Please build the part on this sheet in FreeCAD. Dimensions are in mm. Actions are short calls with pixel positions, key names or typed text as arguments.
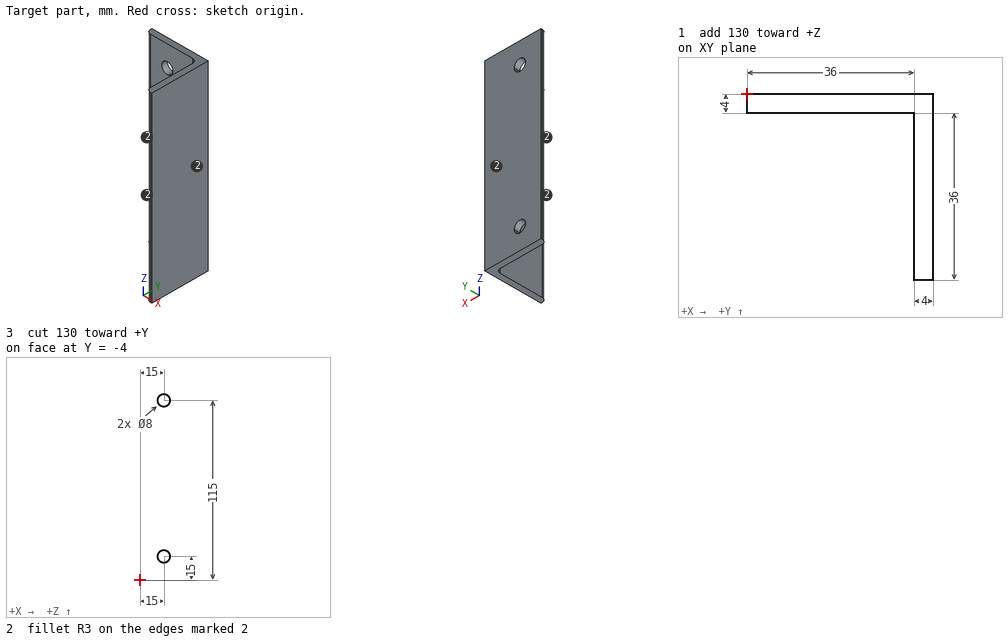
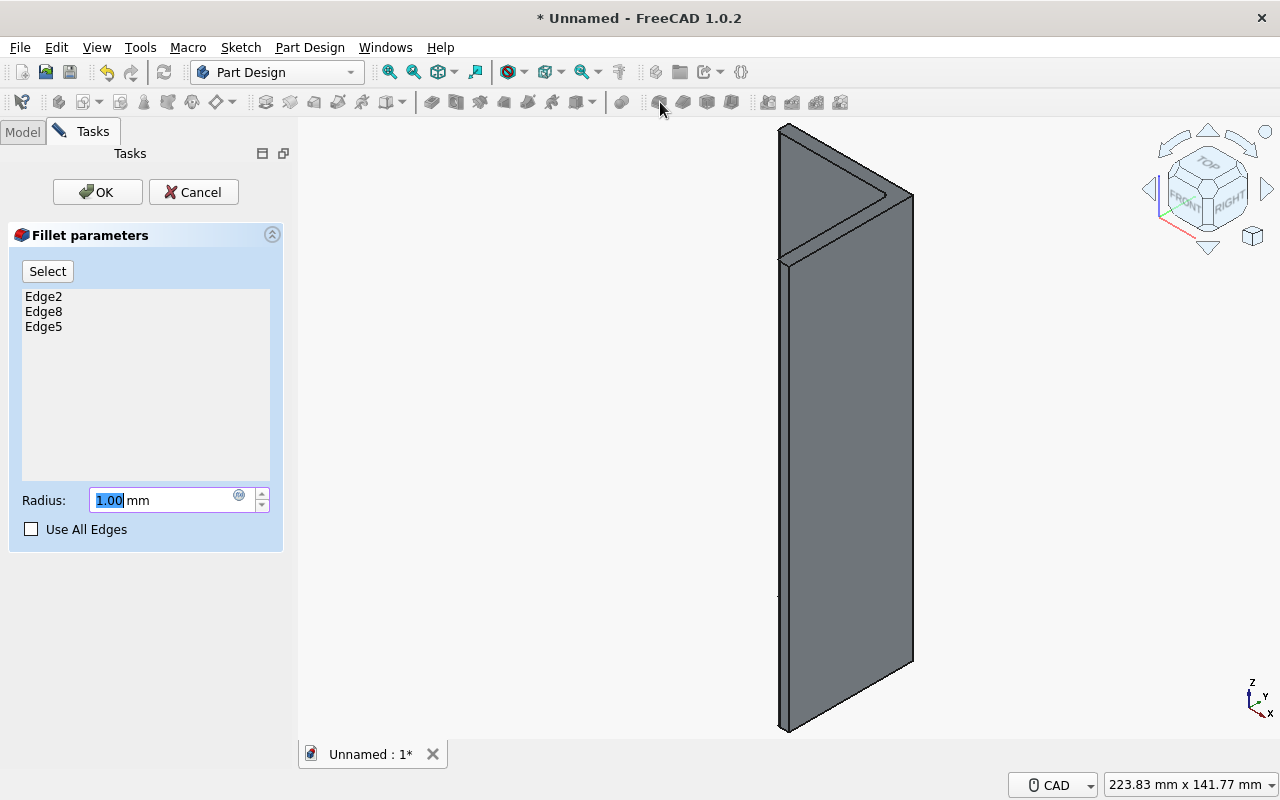
text(3)
key(Tab)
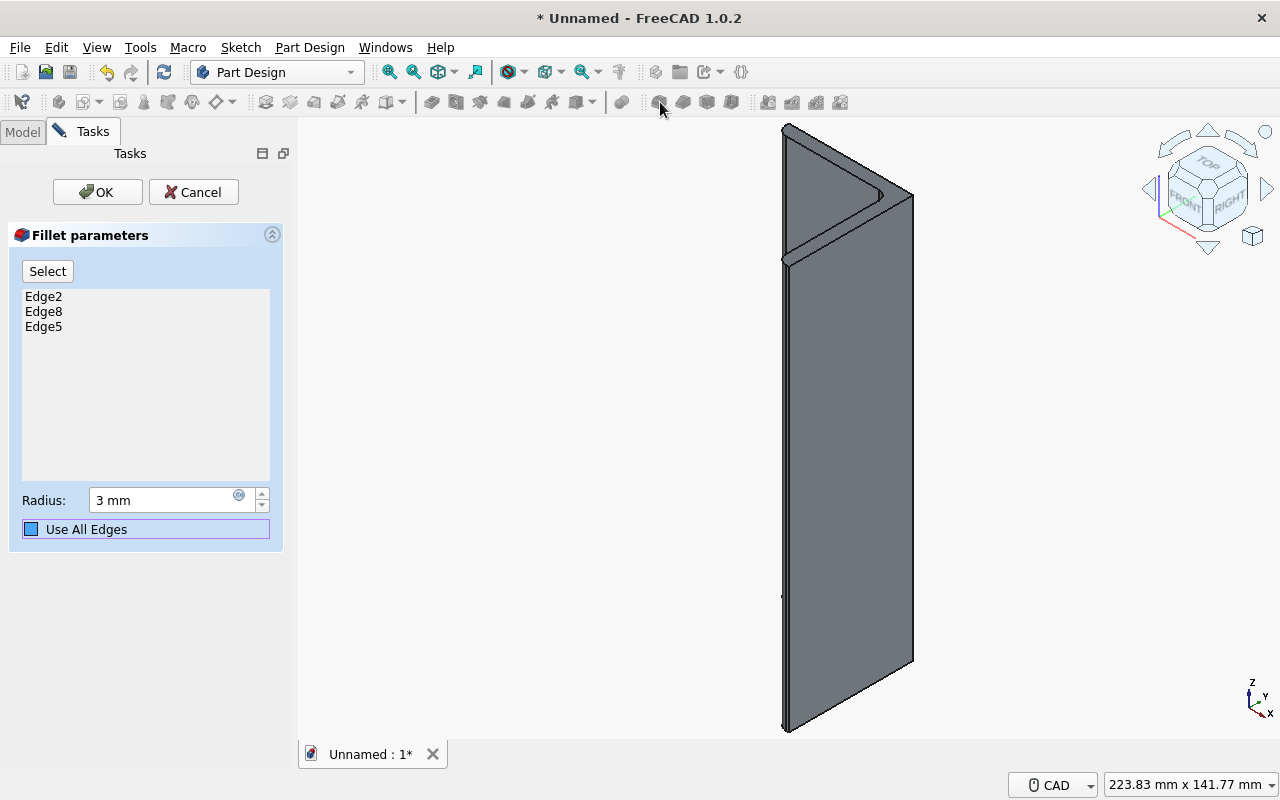
click(98, 192)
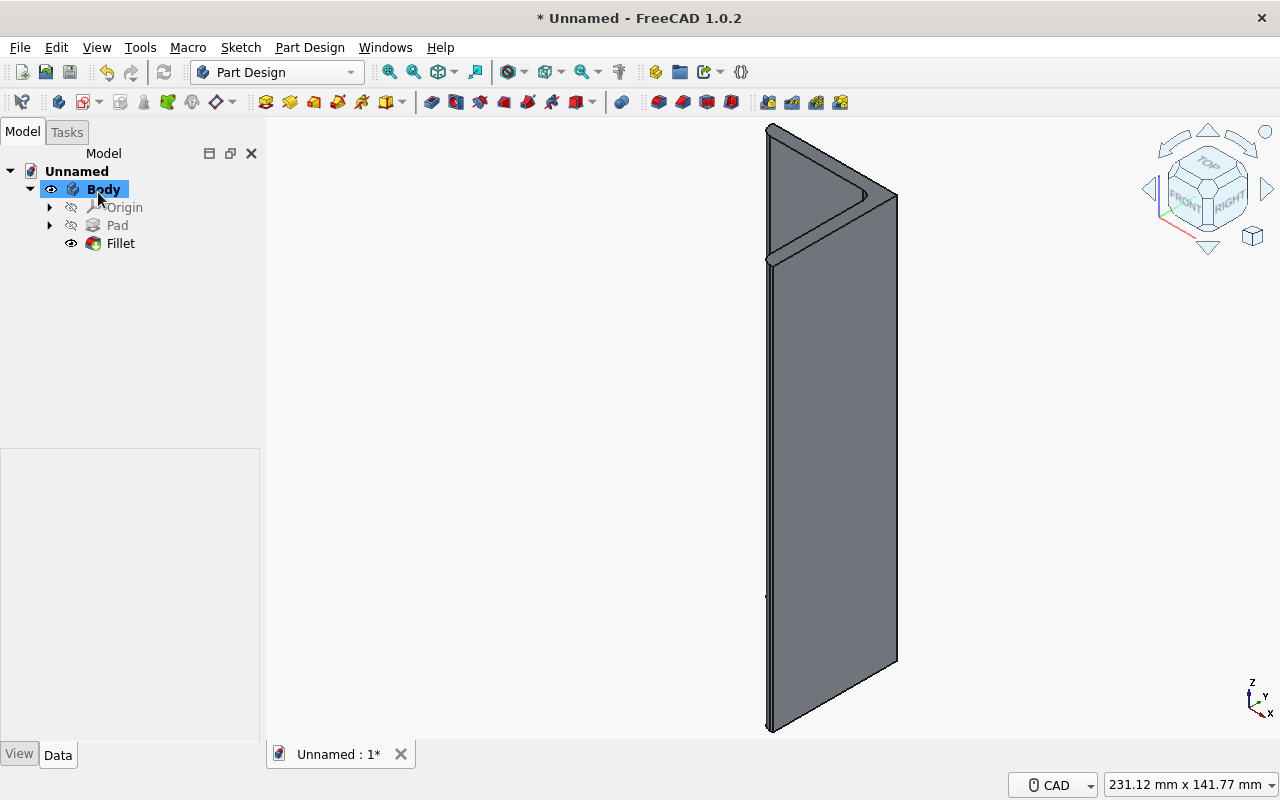
key(1)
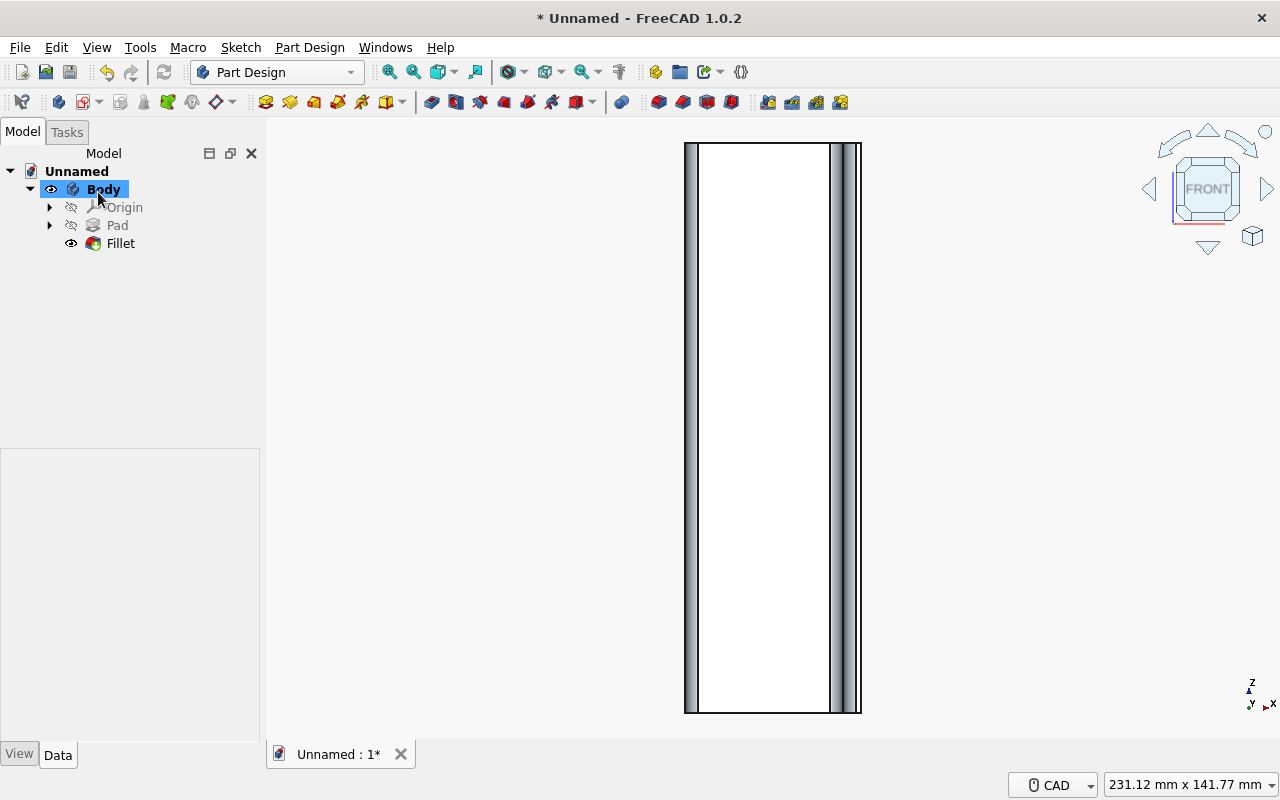
click(764, 264)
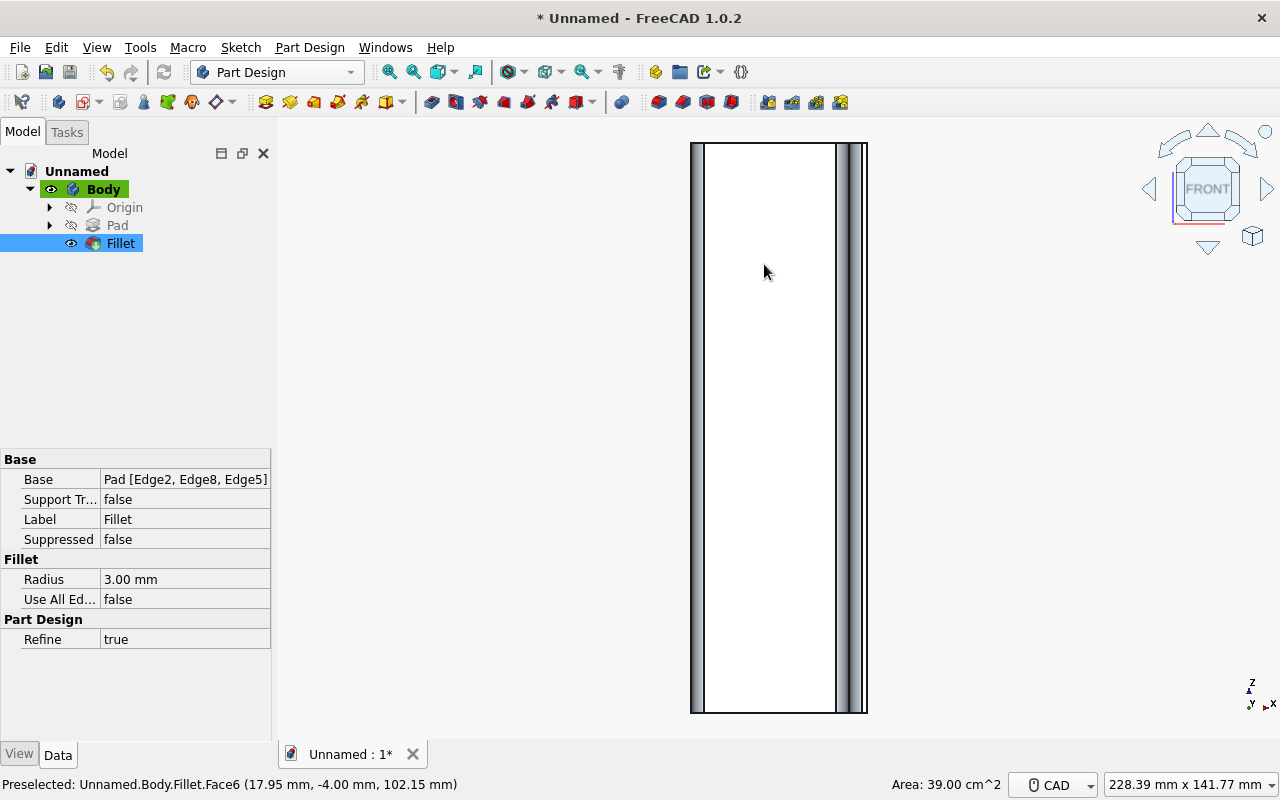
click(84, 102)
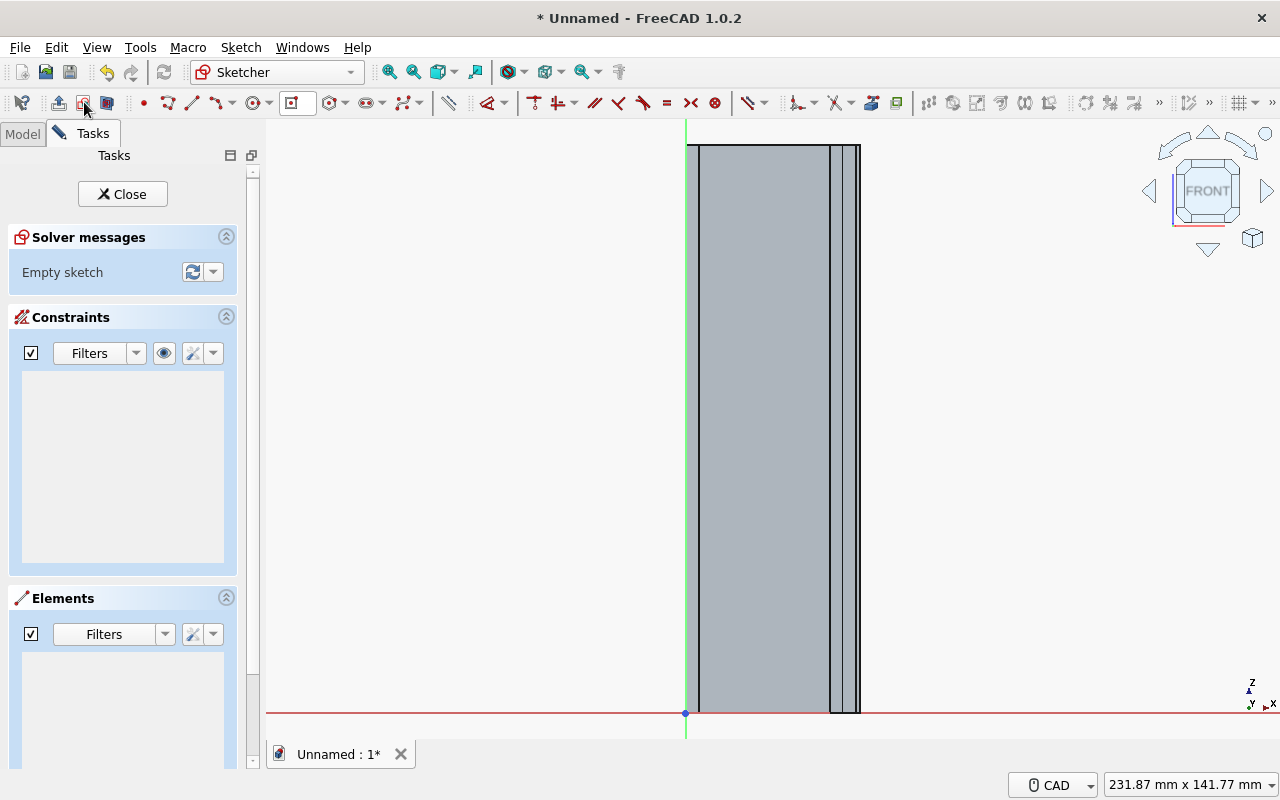
scroll(603, 320, down, 1)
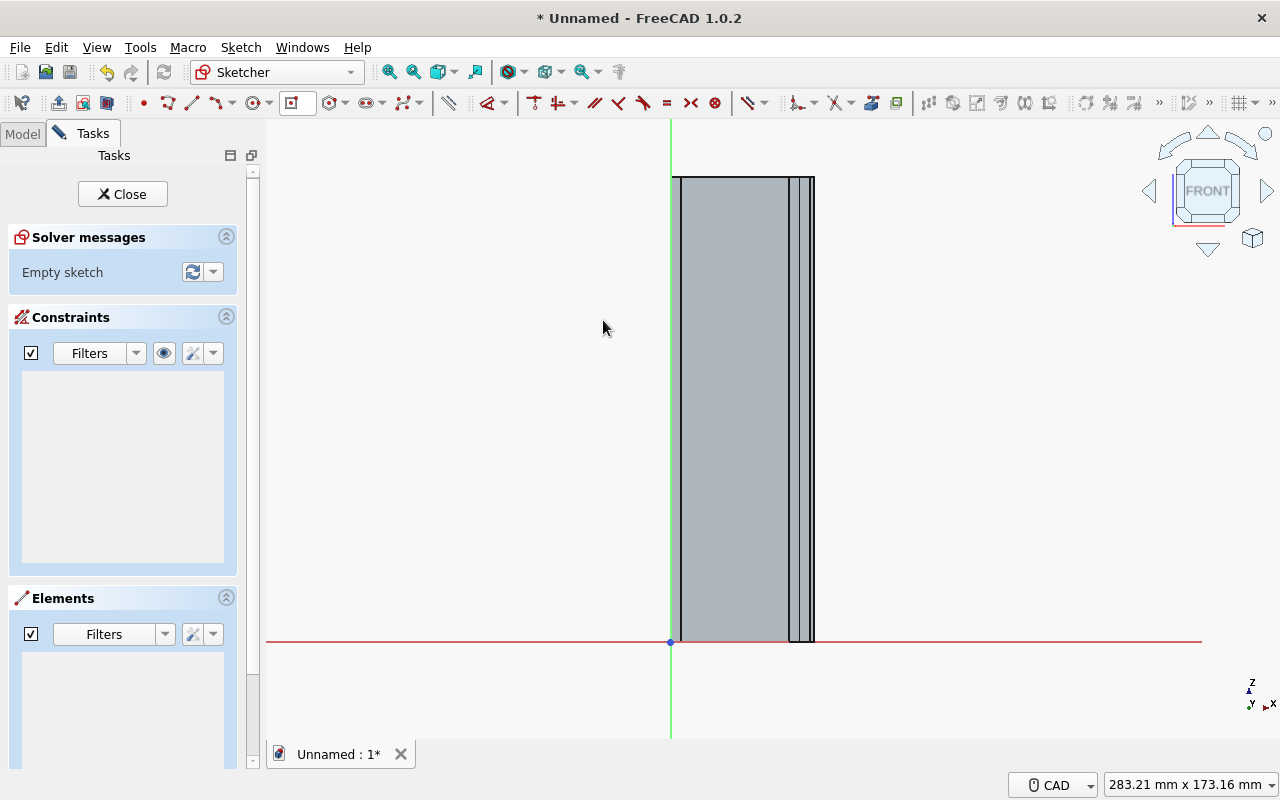
click(254, 104)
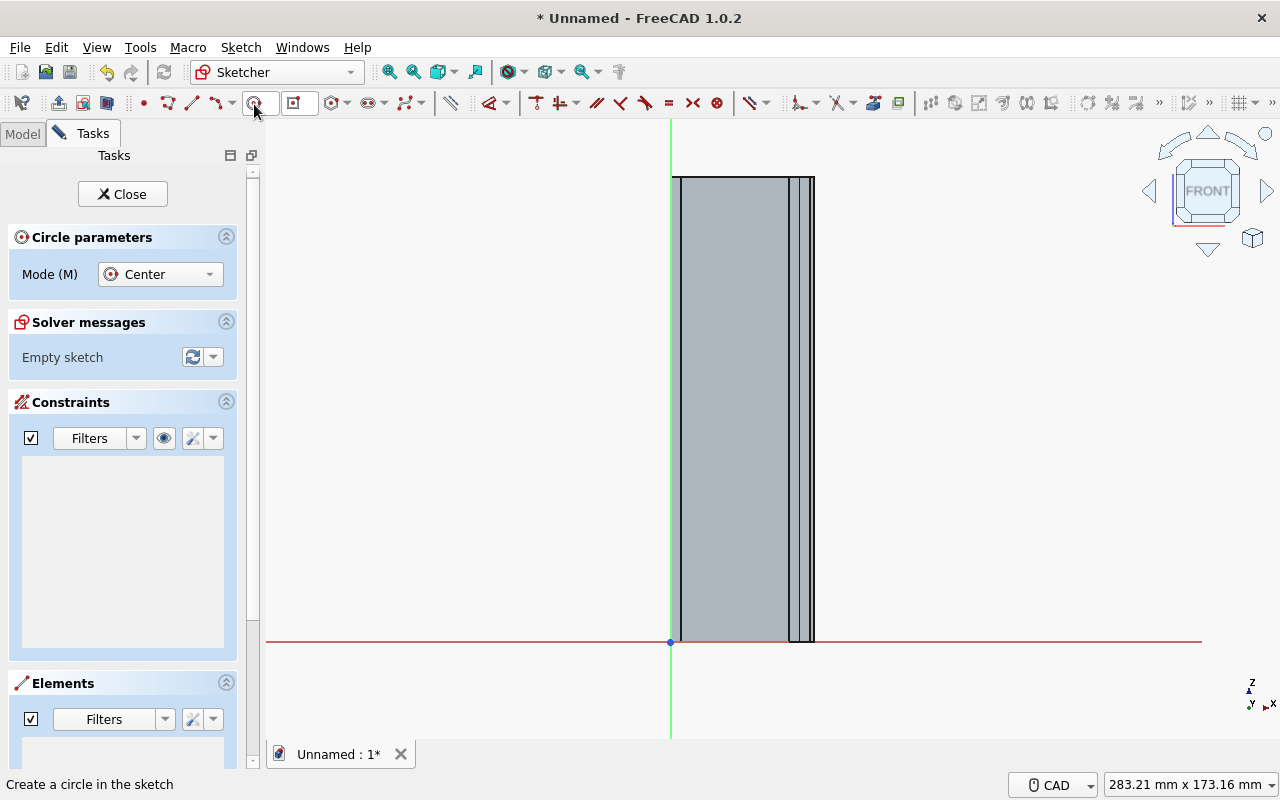
scroll(724, 230, up, 3)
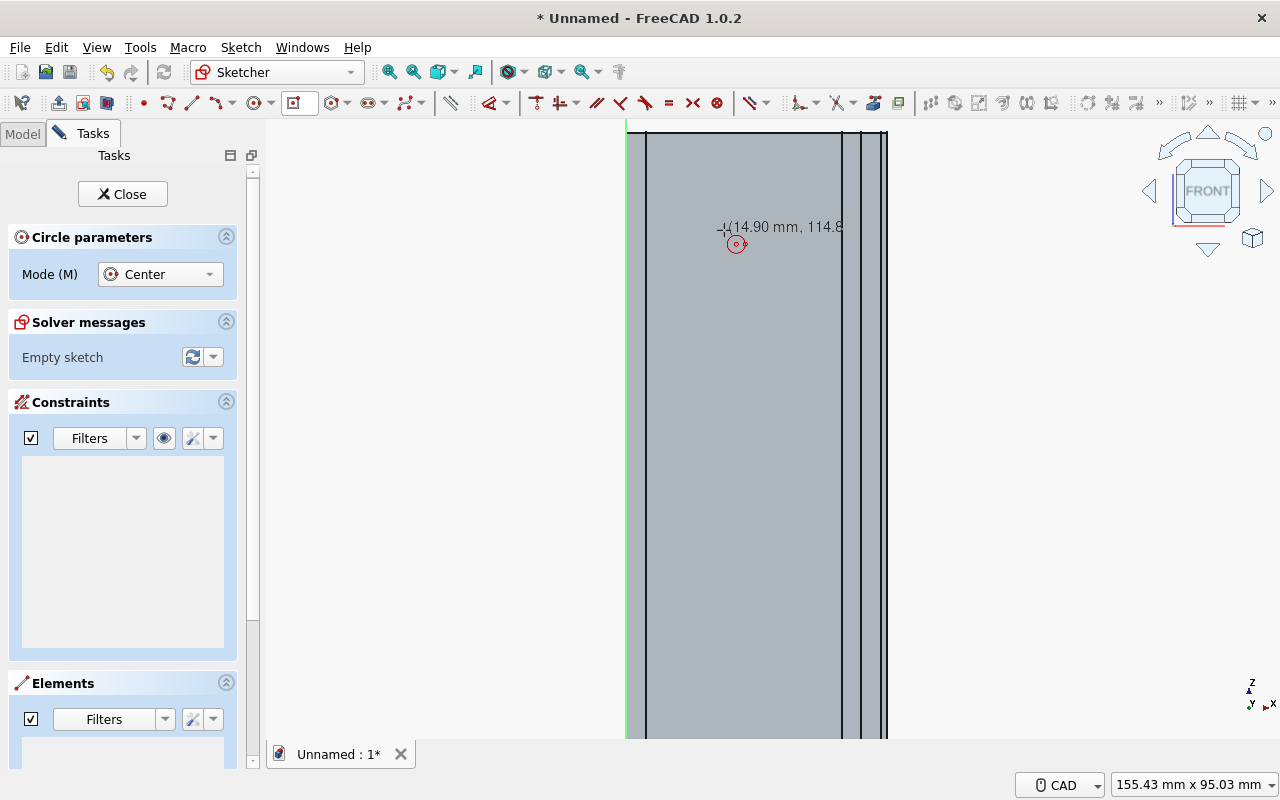
click(724, 230)
move(743, 212)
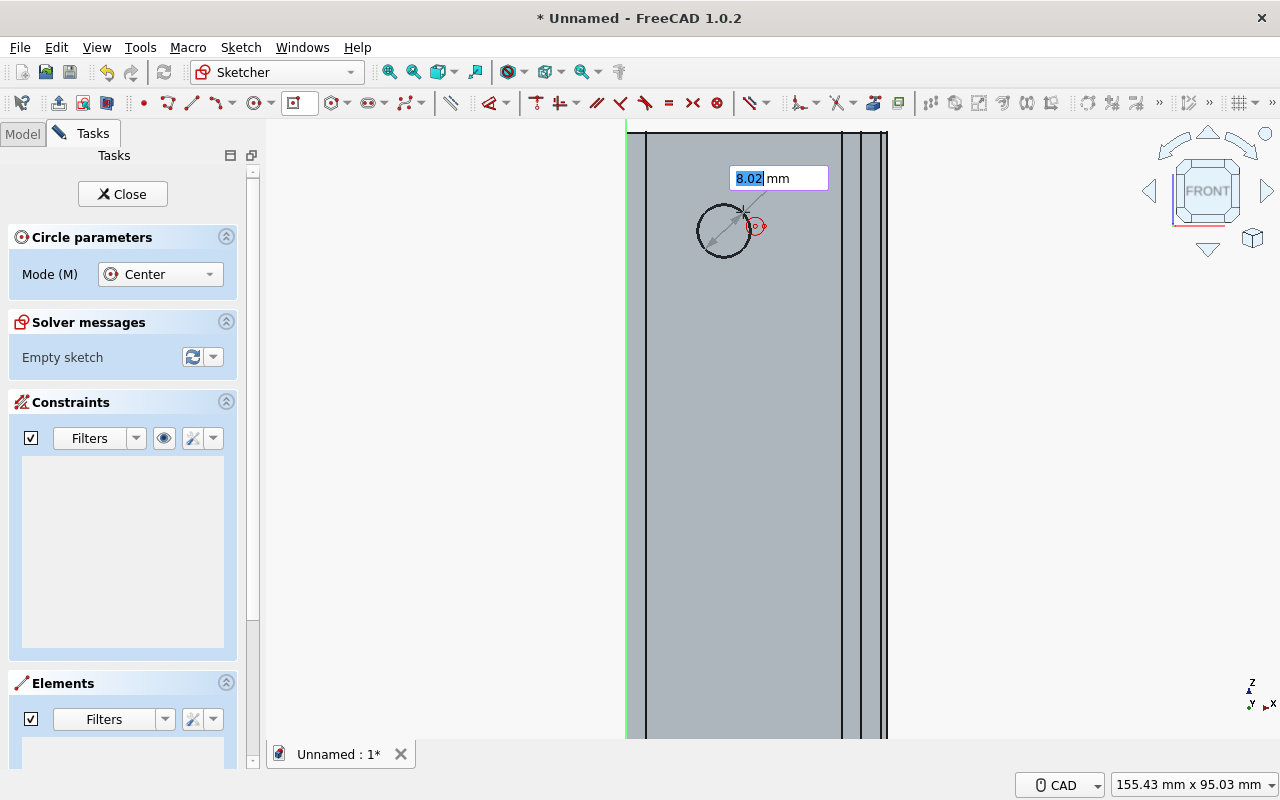
text(8)
key(Return)